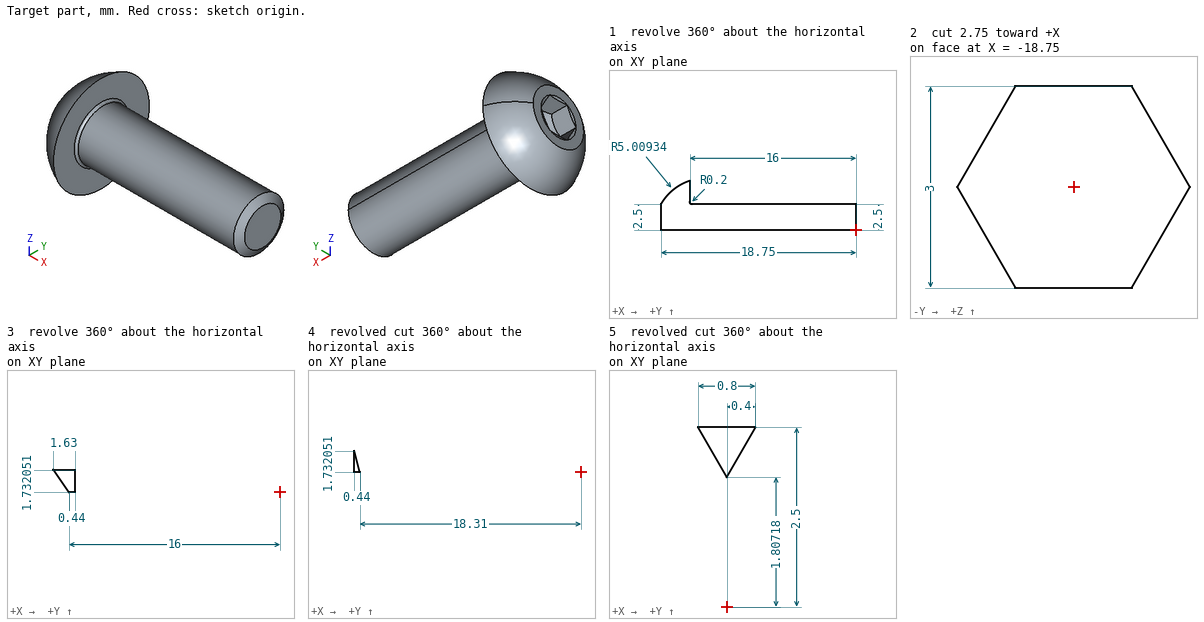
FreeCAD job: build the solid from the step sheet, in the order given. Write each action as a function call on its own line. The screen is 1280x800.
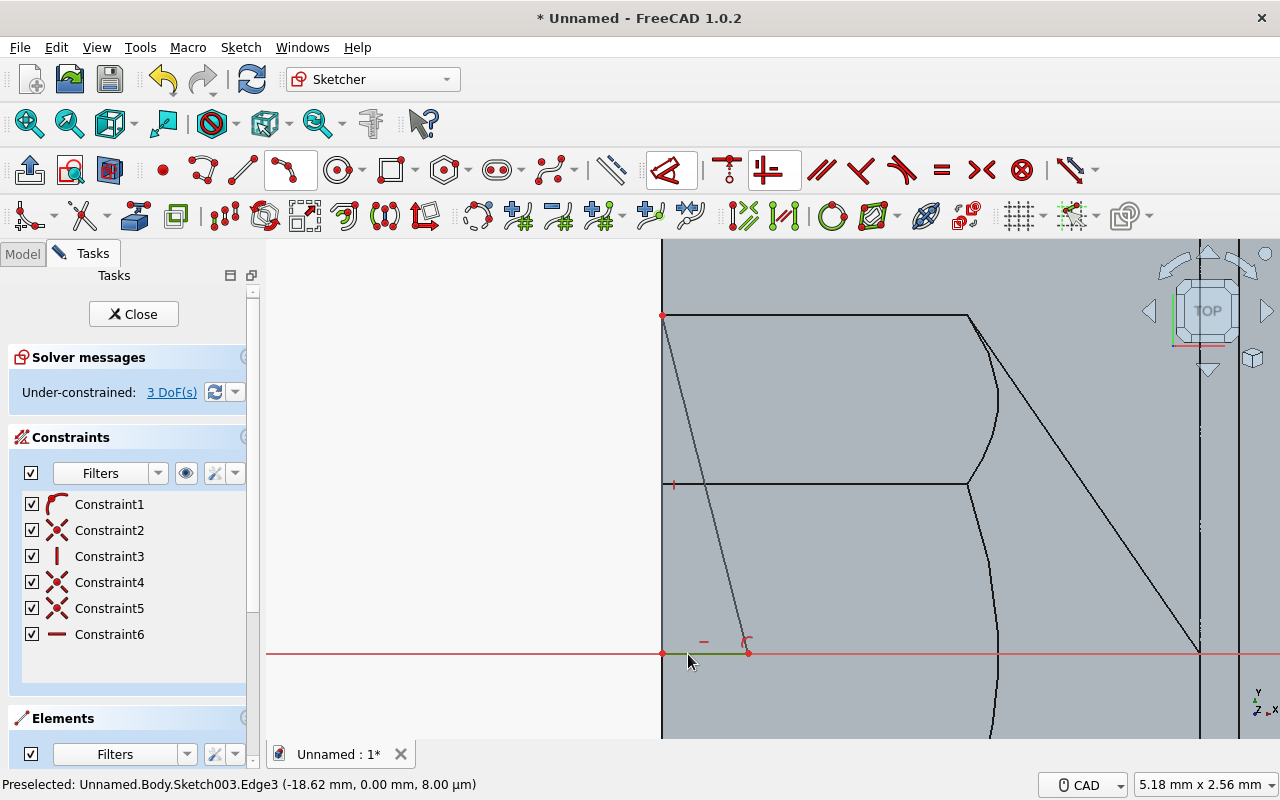
click(692, 170)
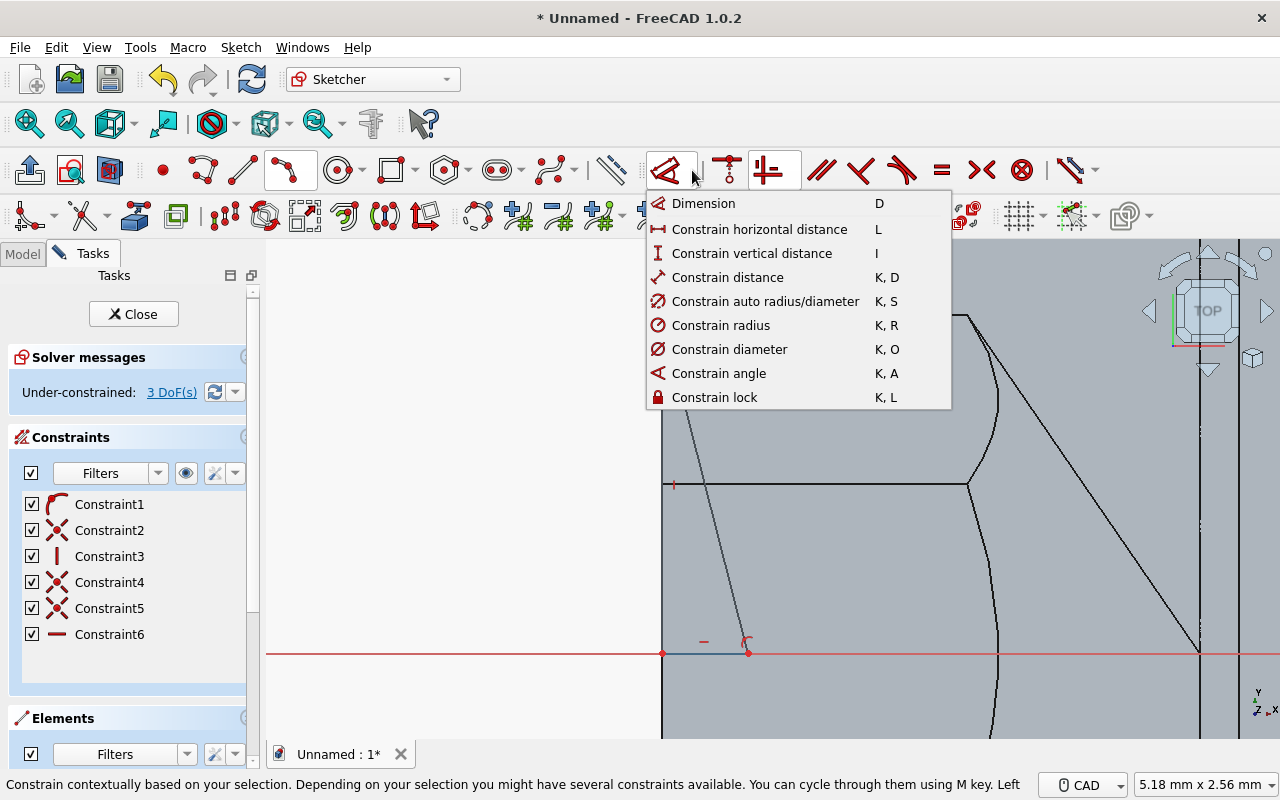
click(799, 229)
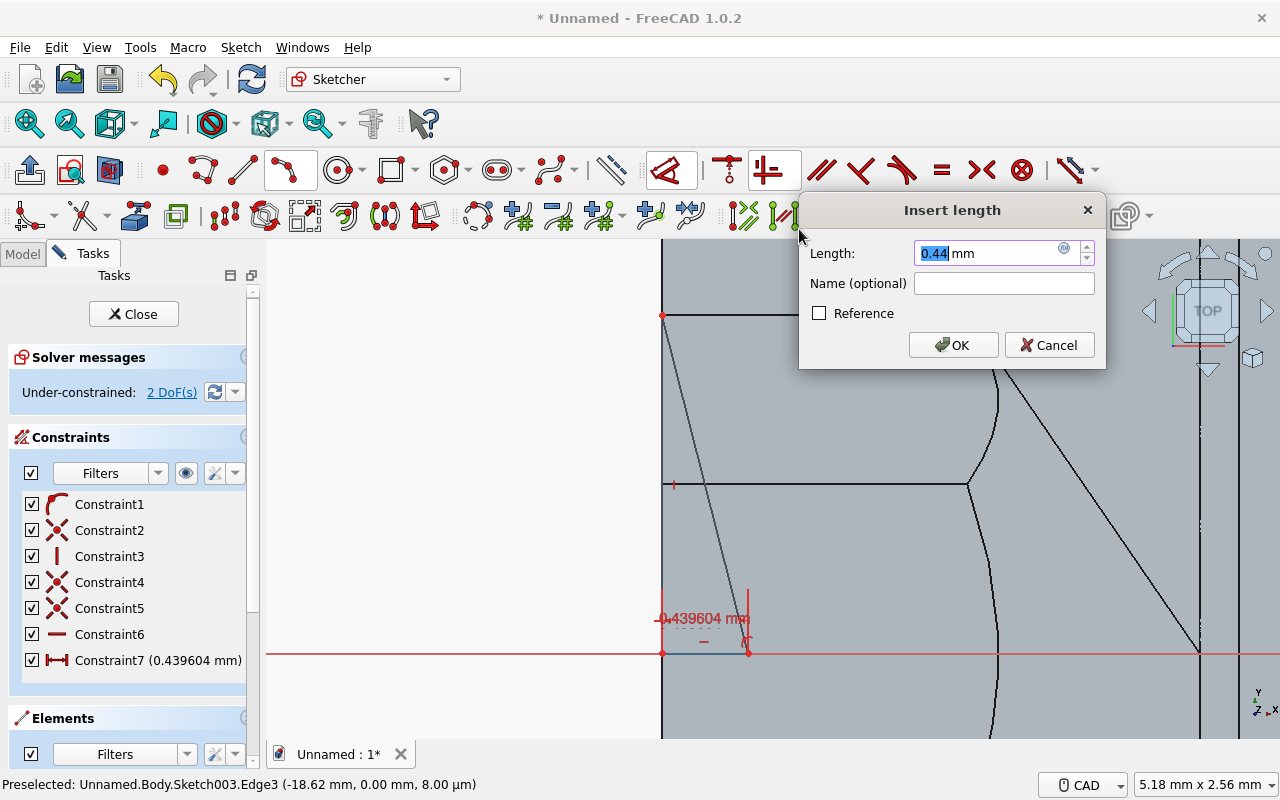
text(0.44)
key(Return)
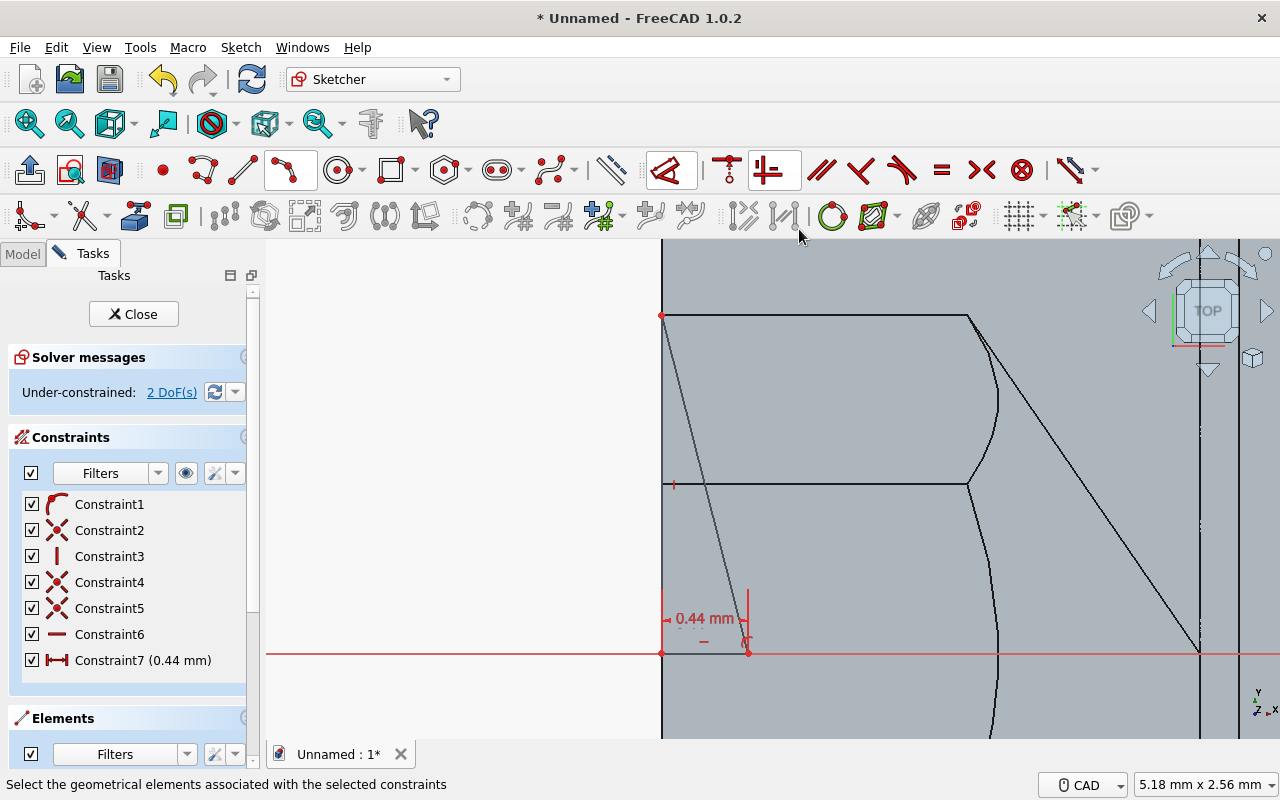
click(748, 654)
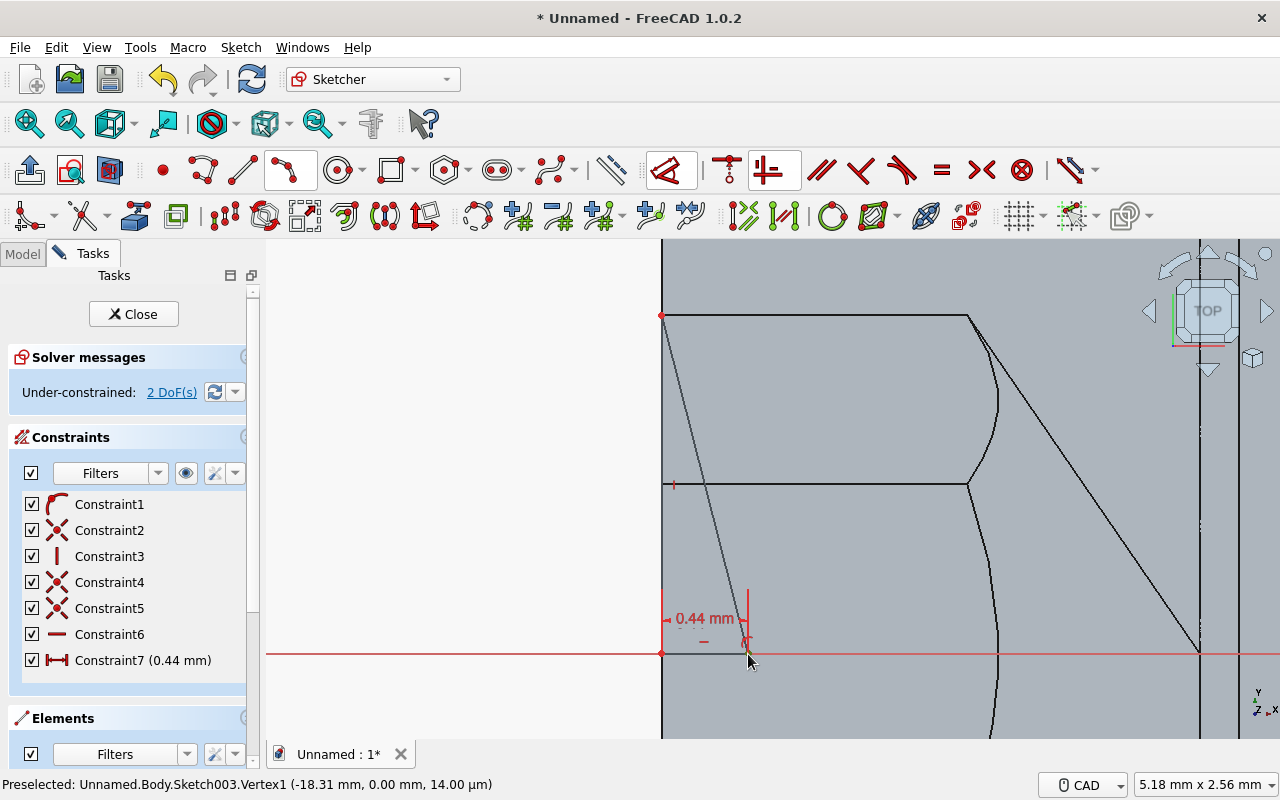
click(692, 170)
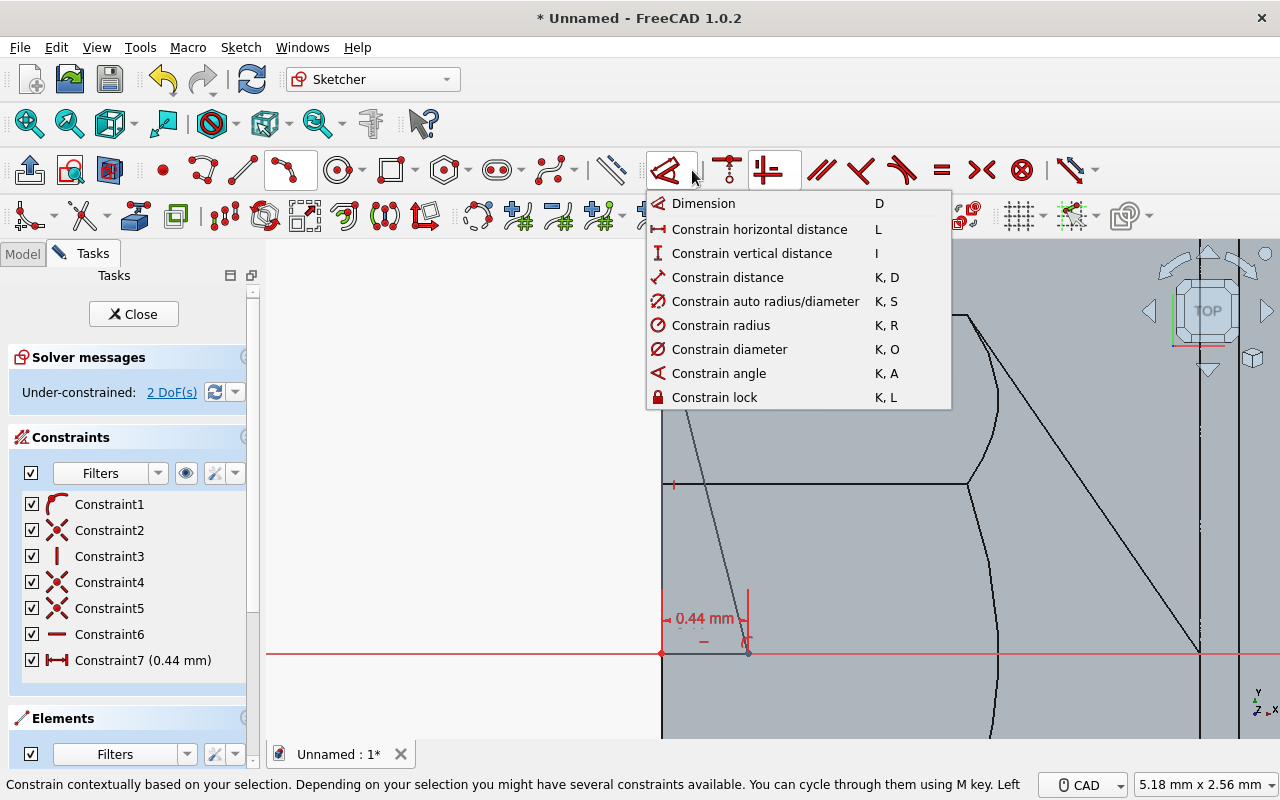
click(799, 229)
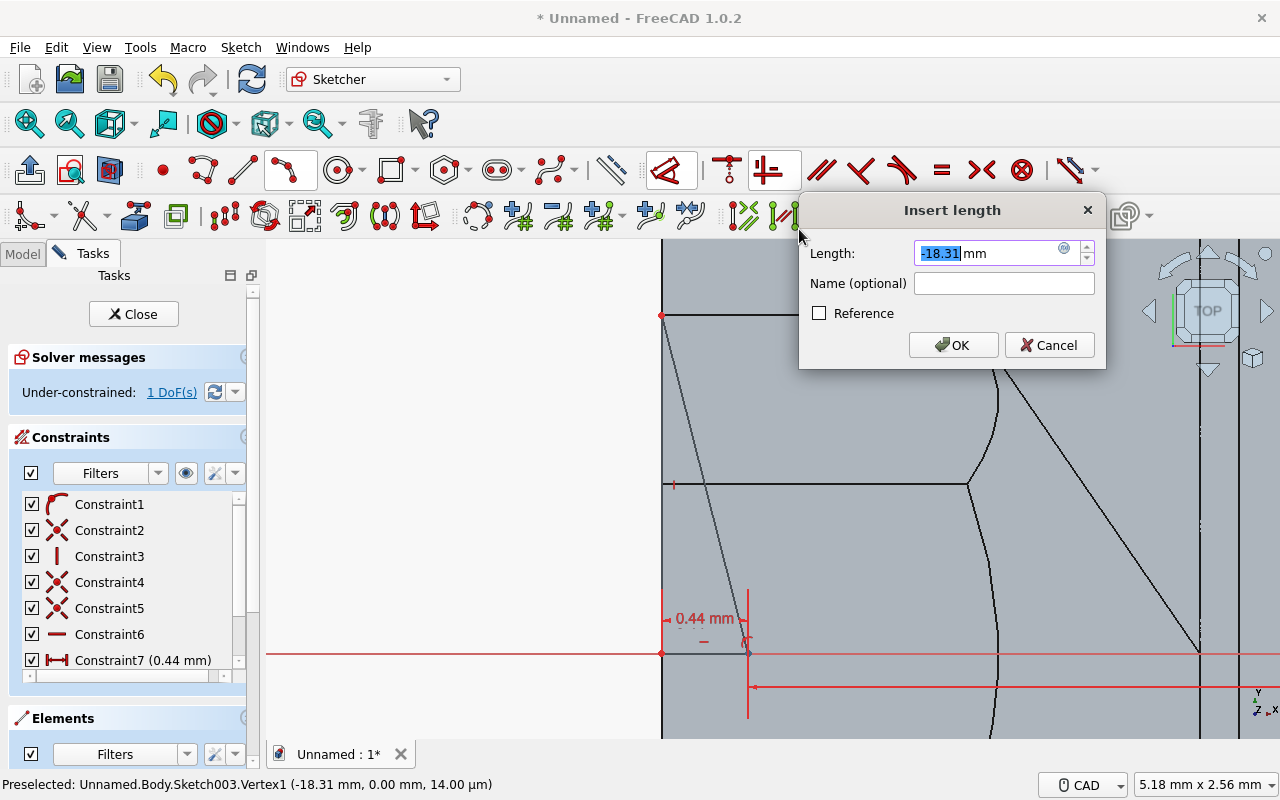
text(-18.31)
key(Return)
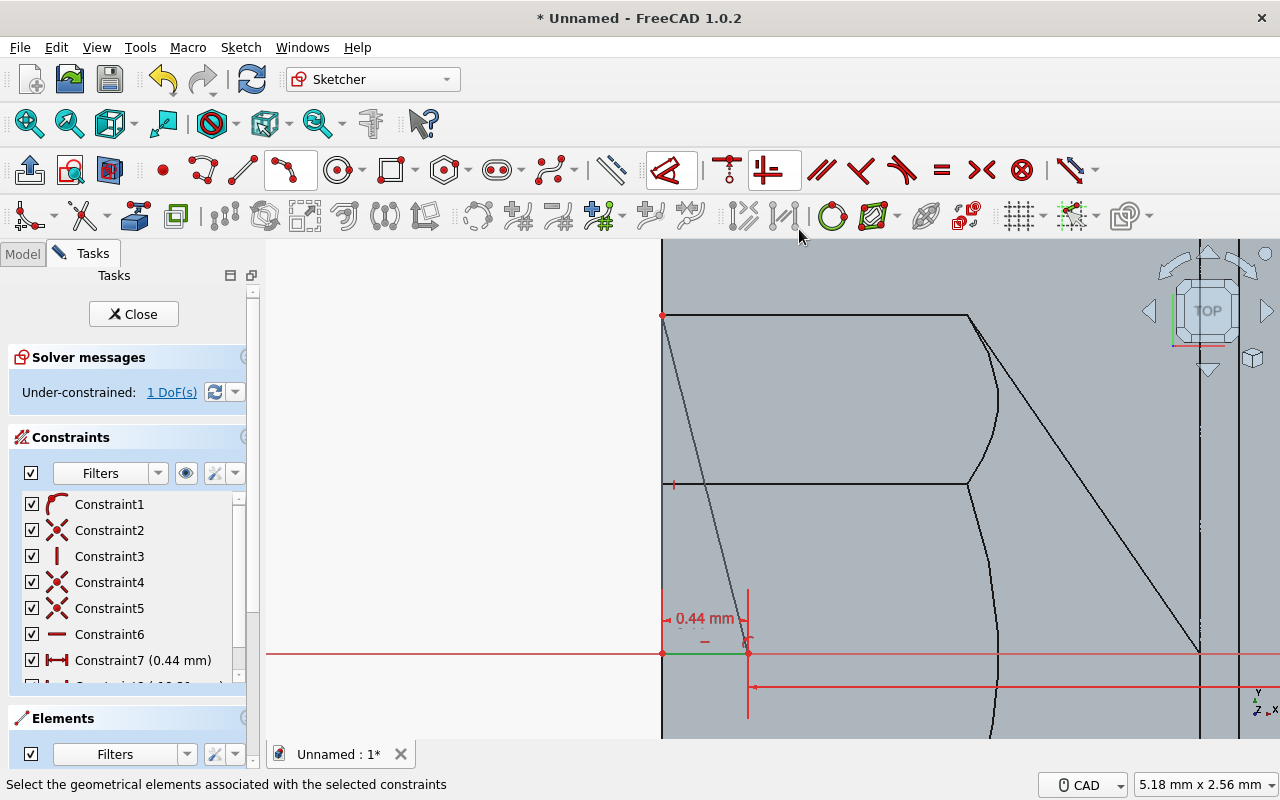
click(662, 417)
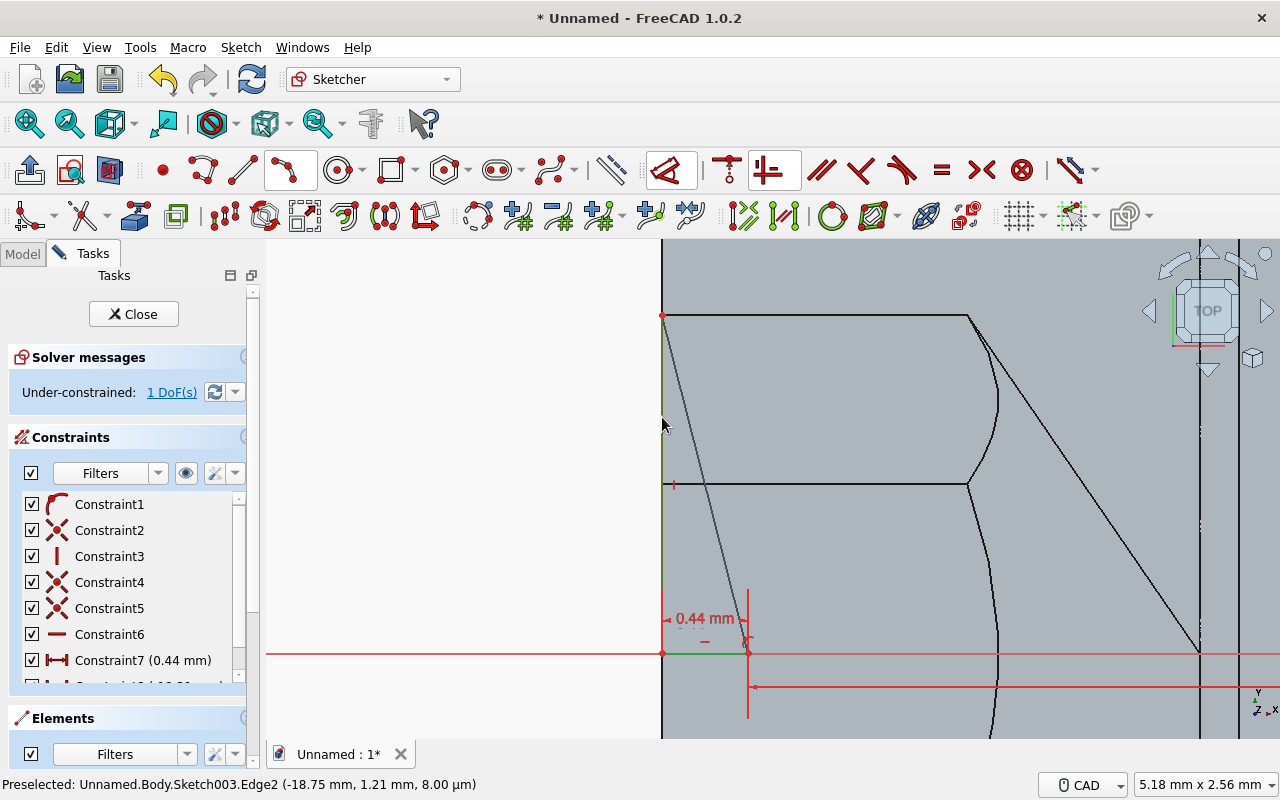
key(i)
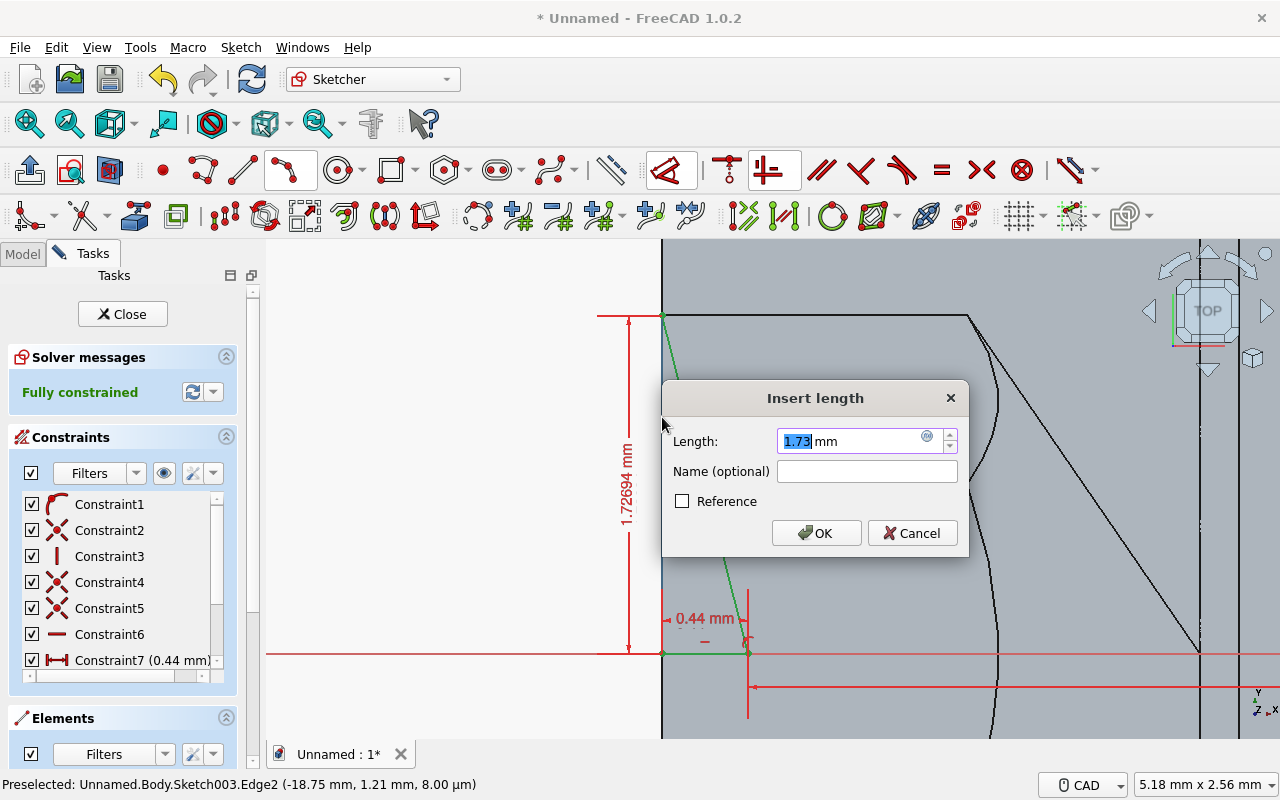
text(1.732051)
key(Return)